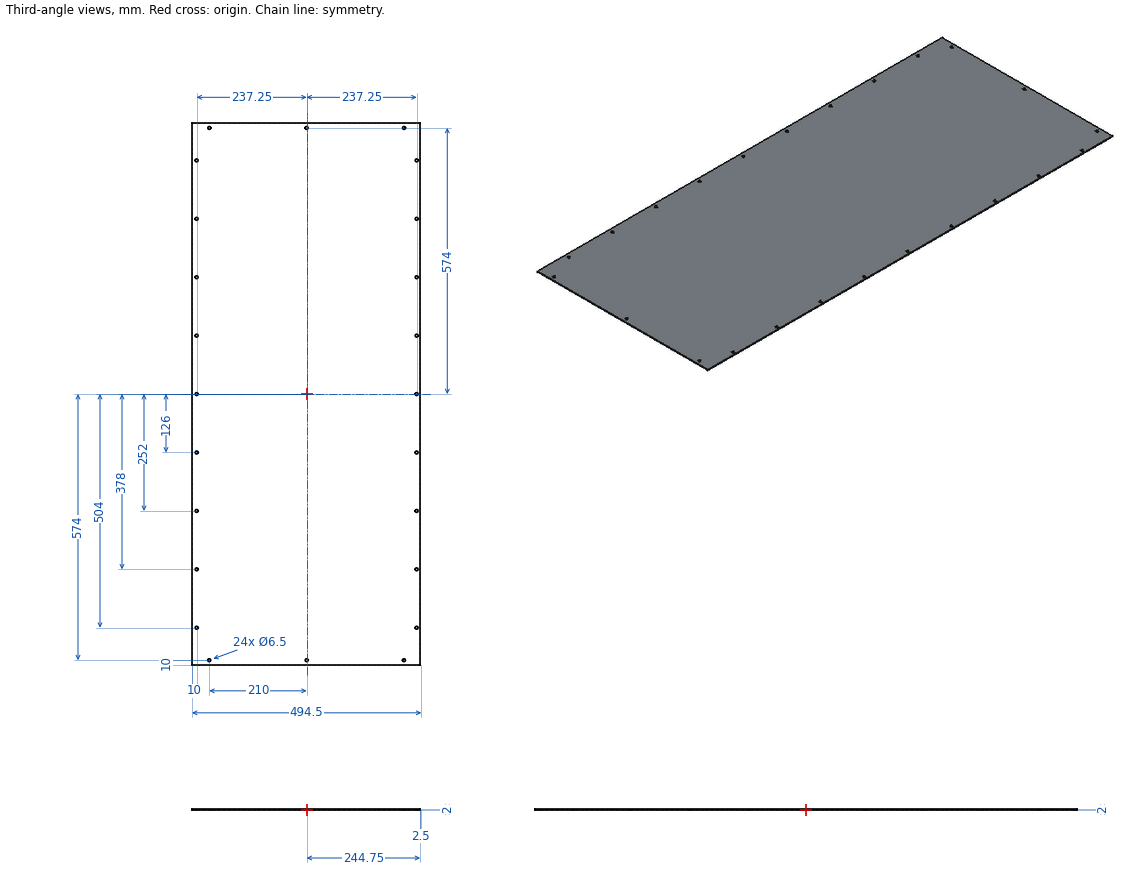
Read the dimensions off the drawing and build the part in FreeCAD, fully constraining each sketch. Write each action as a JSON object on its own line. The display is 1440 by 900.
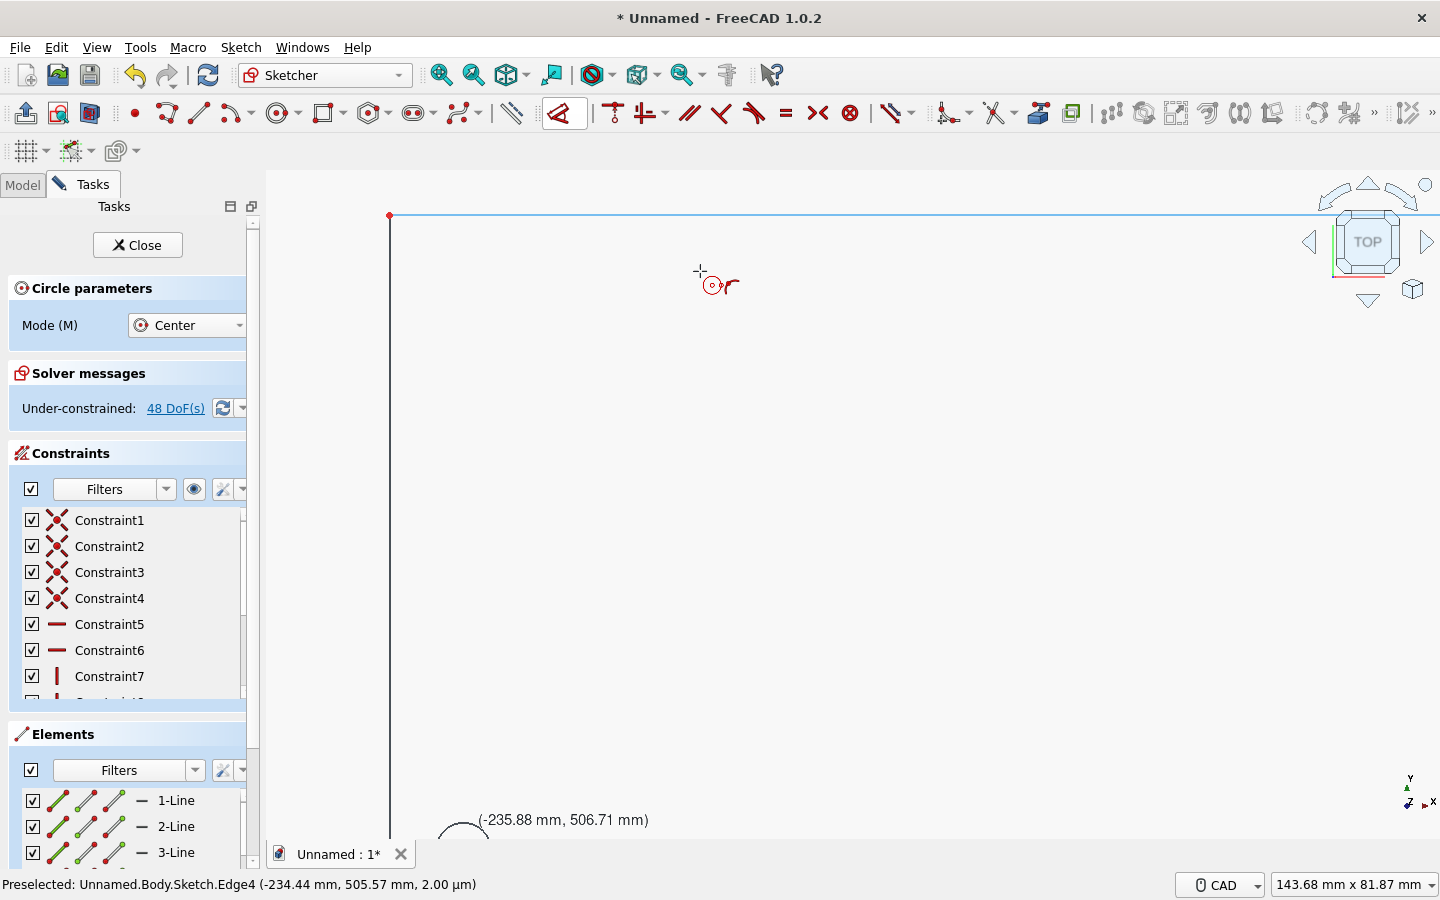
{"action": "scroll", "coordinate": [700, 271], "scroll_direction": "down", "scroll_amount": 15}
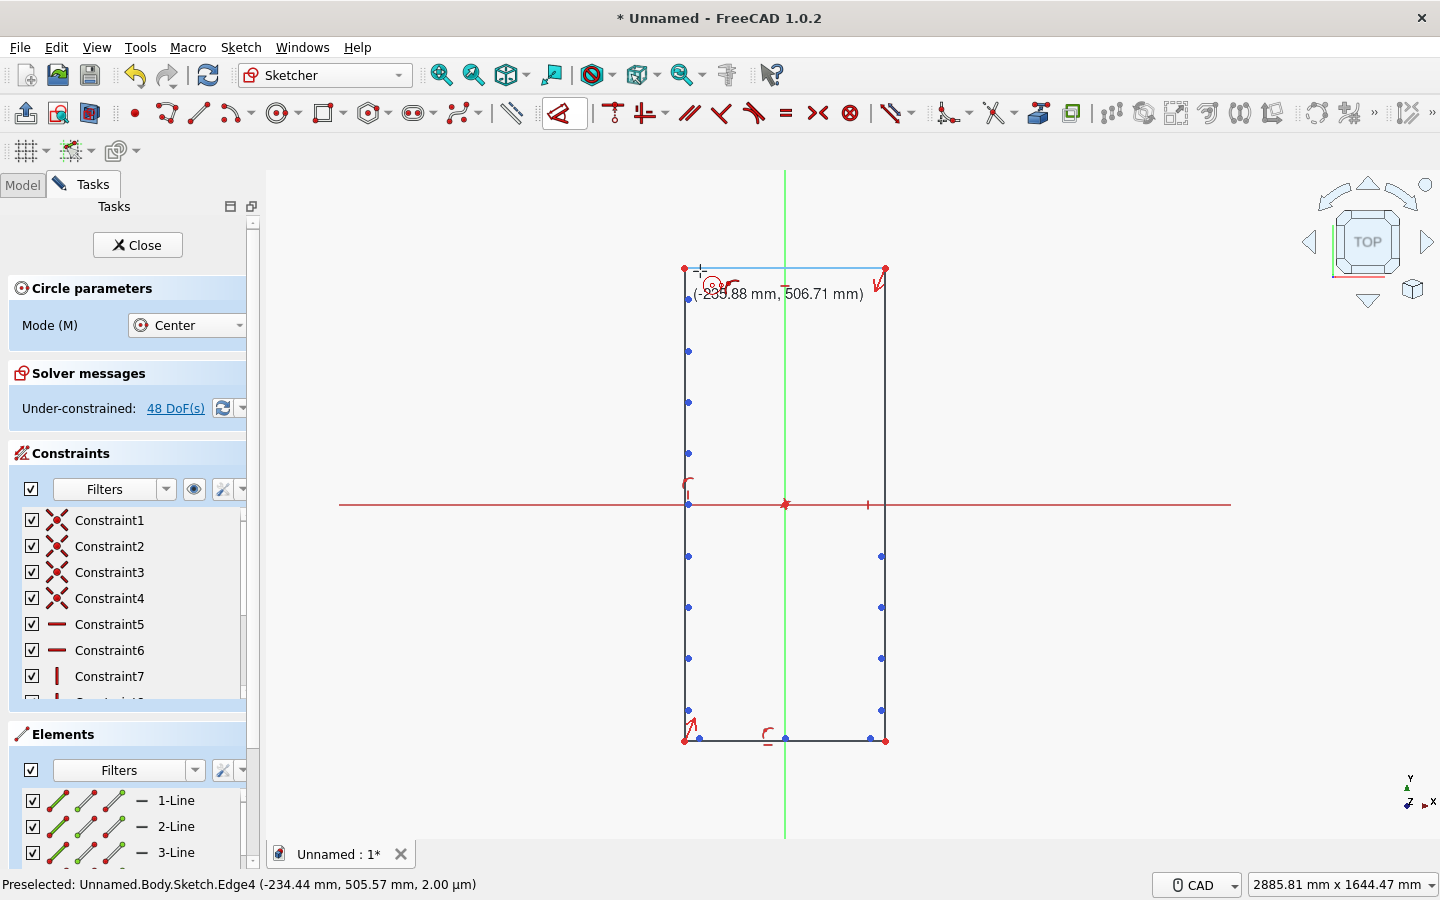
{"action": "scroll", "coordinate": [700, 271], "scroll_direction": "up", "scroll_amount": 7}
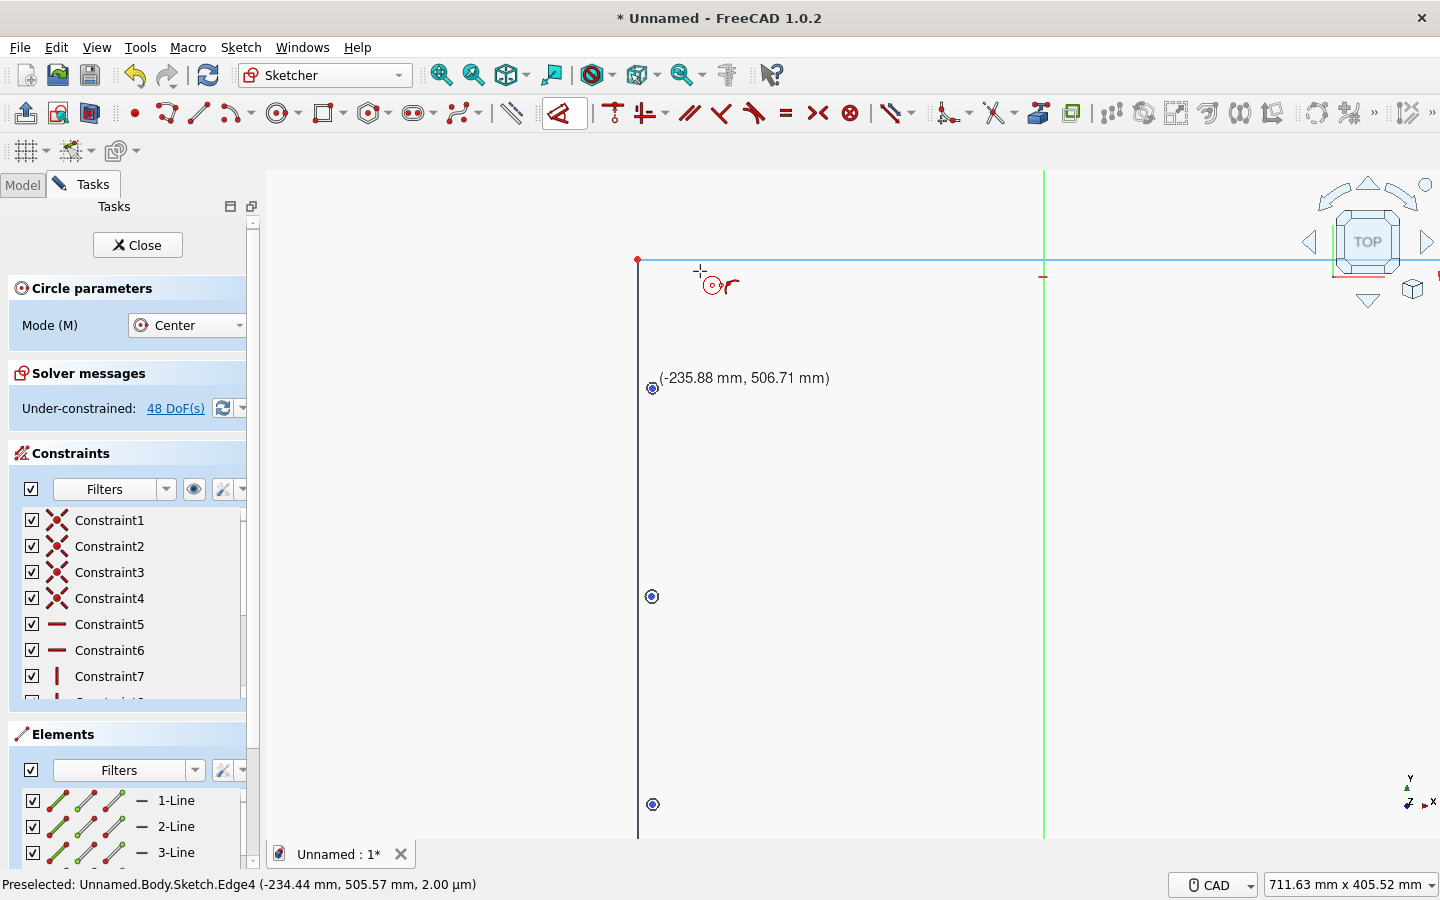
{"action": "left_click", "coordinate": [697, 272]}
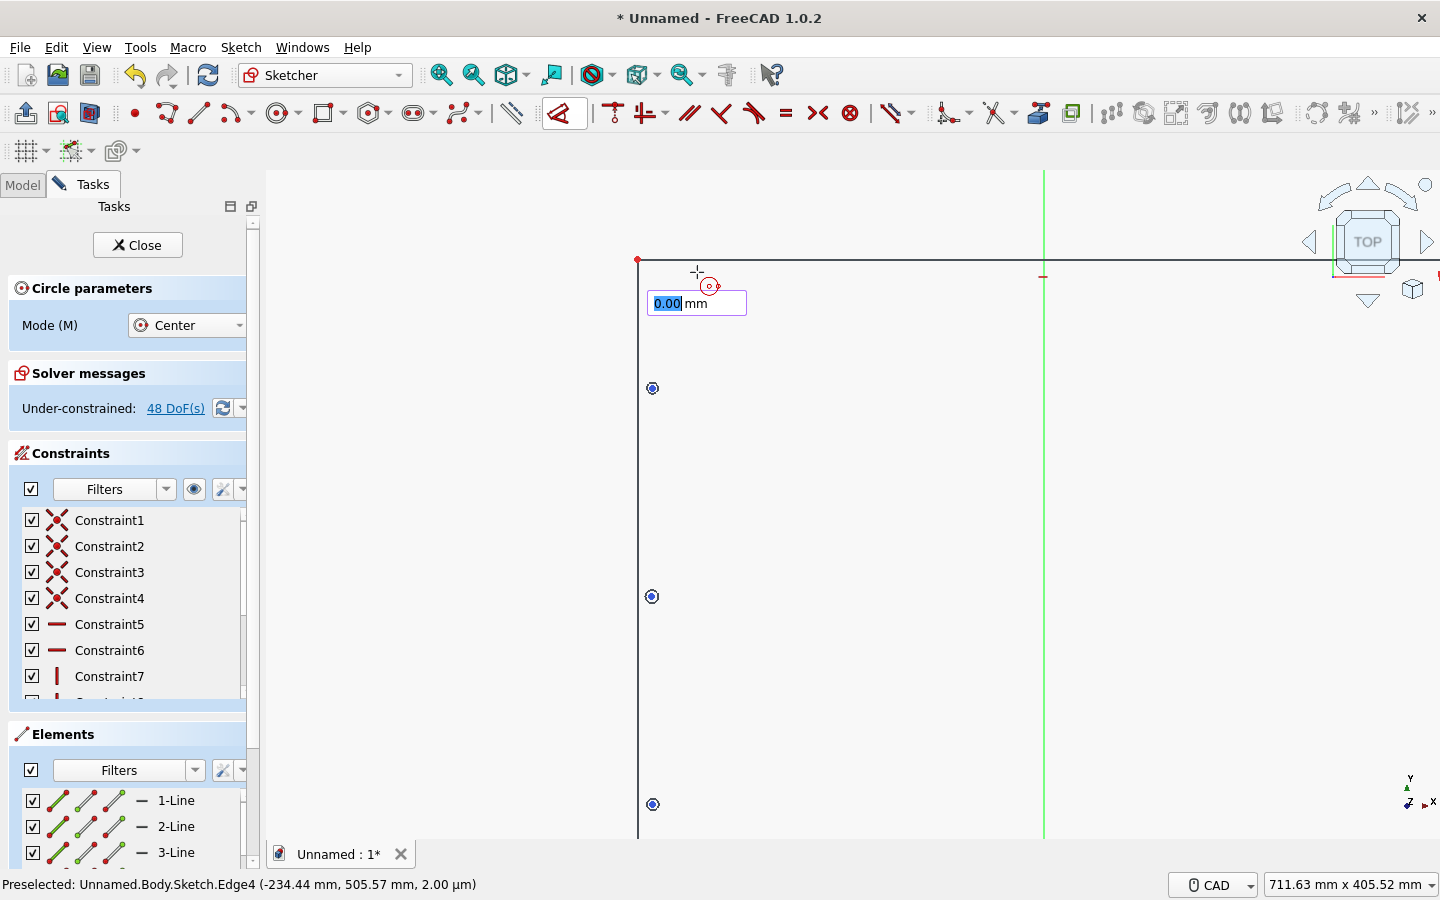
{"action": "scroll", "coordinate": [701, 276], "scroll_direction": "up", "scroll_amount": 6}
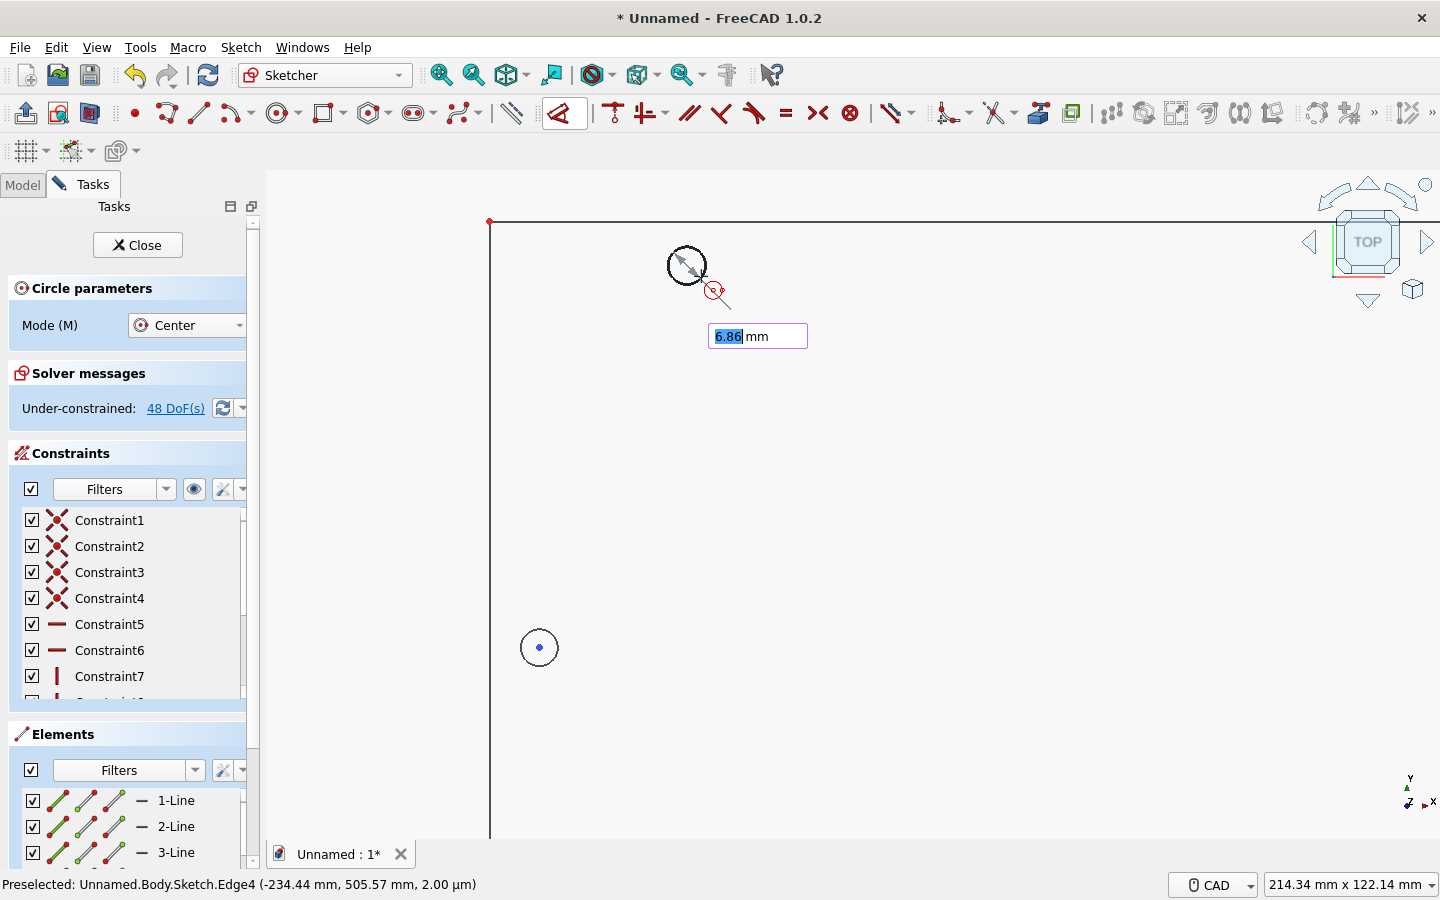
{"action": "left_click", "coordinate": [701, 275]}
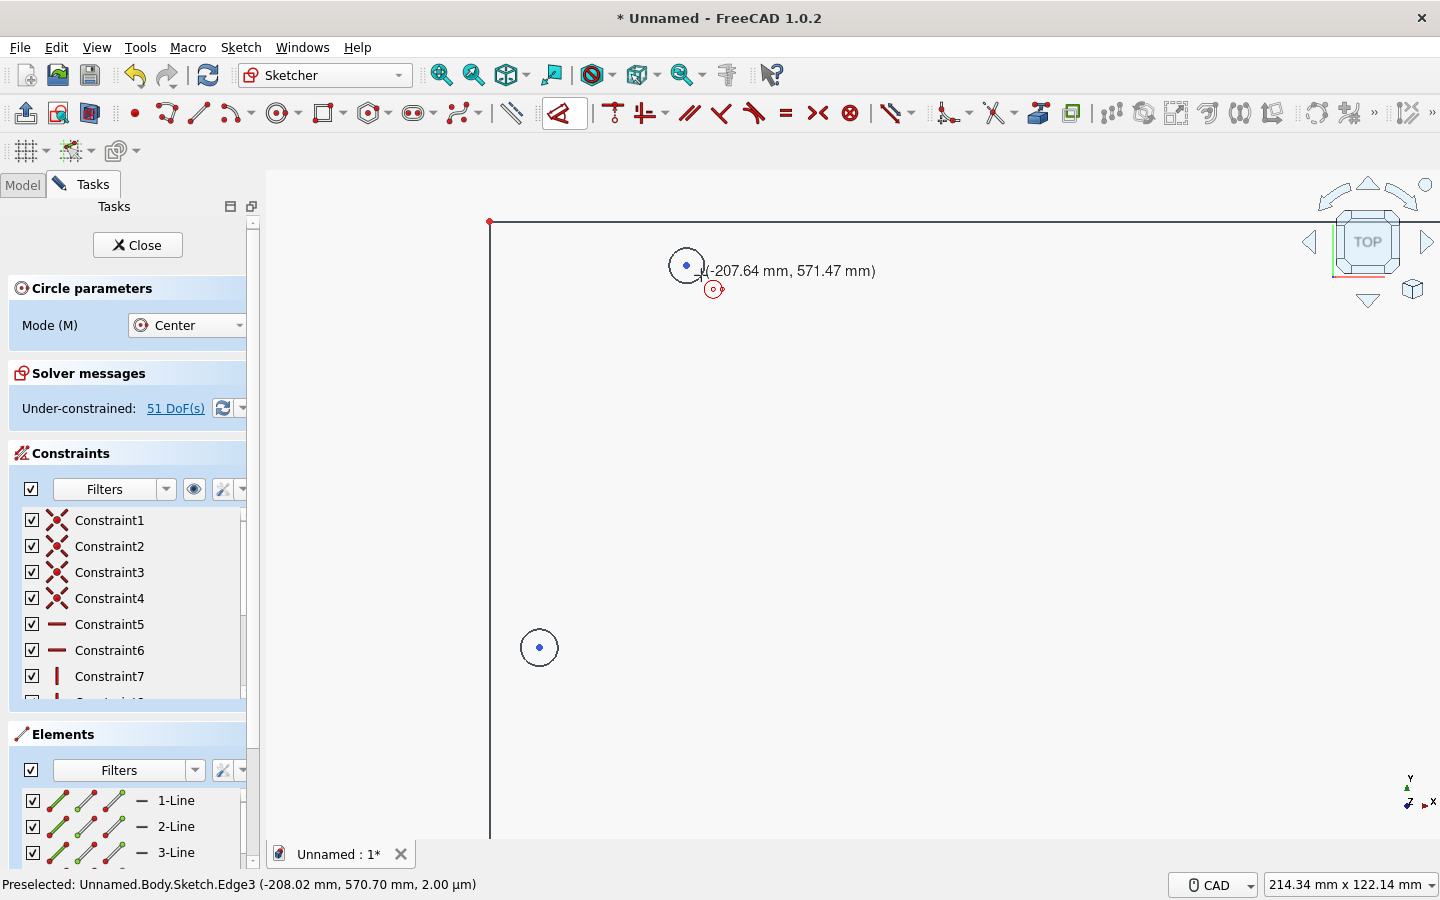
{"action": "scroll", "coordinate": [700, 272], "scroll_direction": "down", "scroll_amount": 13}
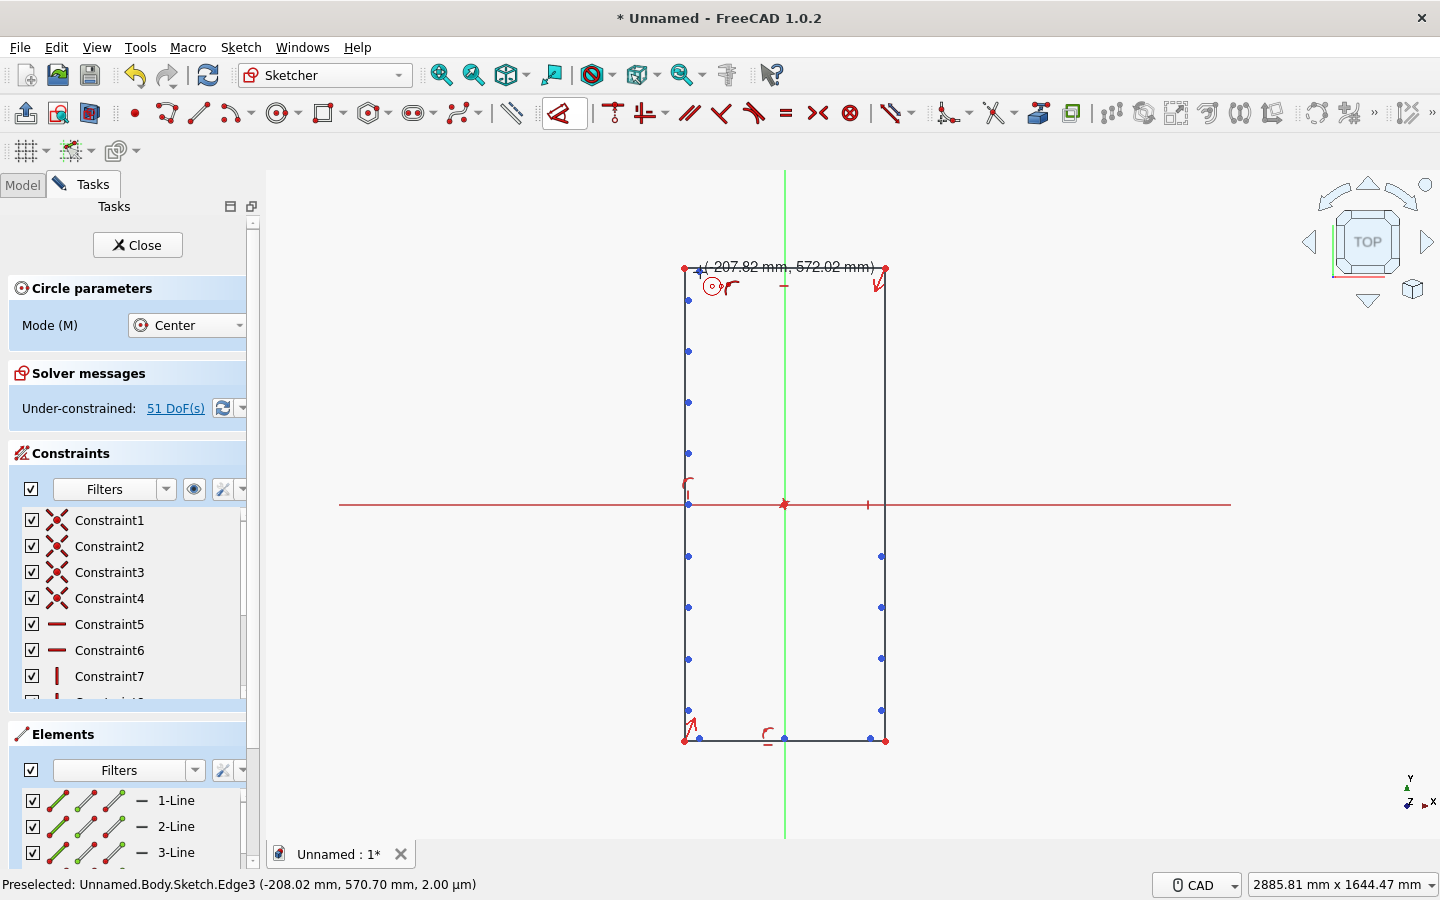
{"action": "scroll", "coordinate": [881, 505], "scroll_direction": "up", "scroll_amount": 15}